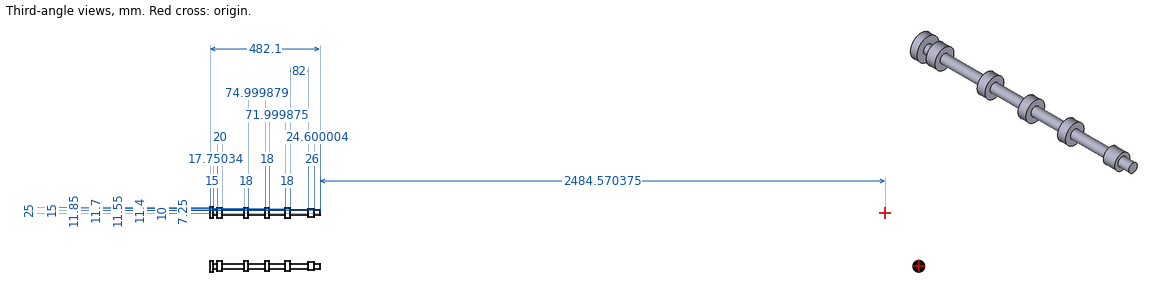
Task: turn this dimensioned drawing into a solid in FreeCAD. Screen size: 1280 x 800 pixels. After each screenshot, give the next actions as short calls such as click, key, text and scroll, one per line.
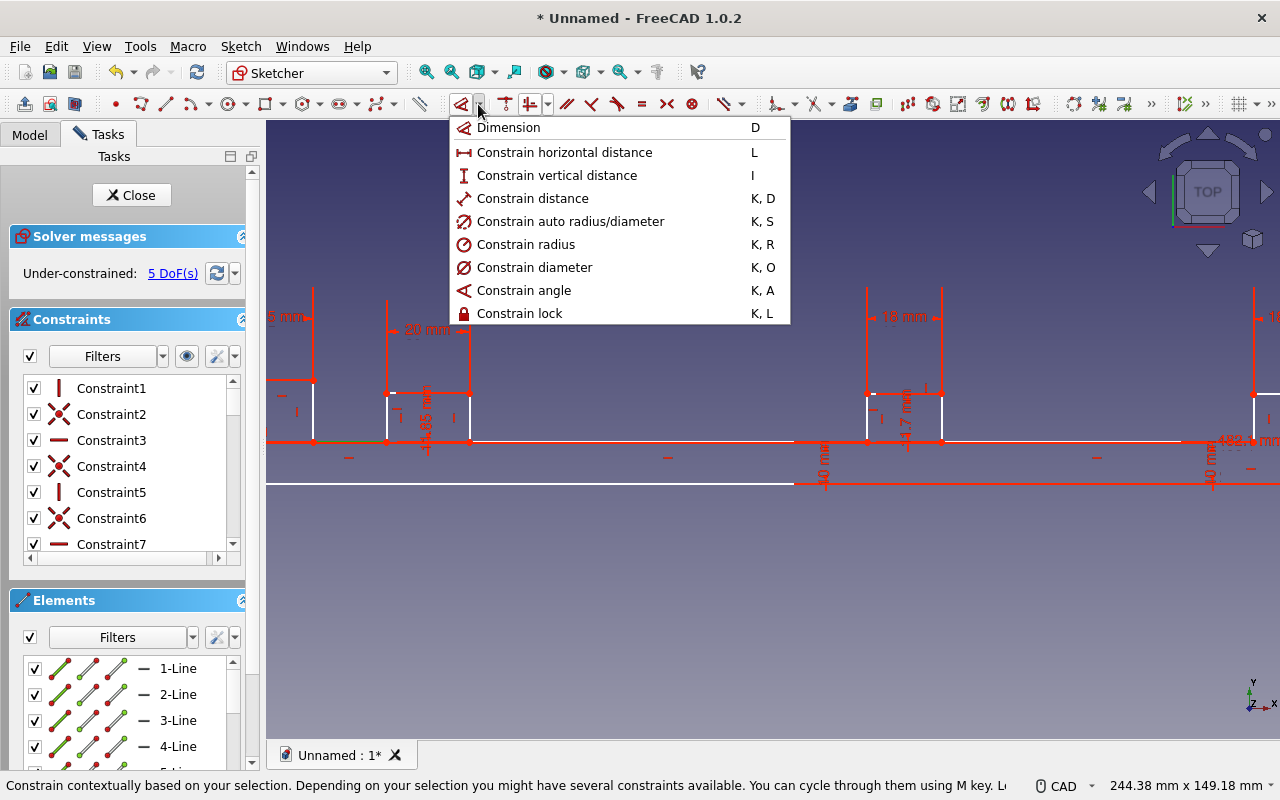
click(620, 152)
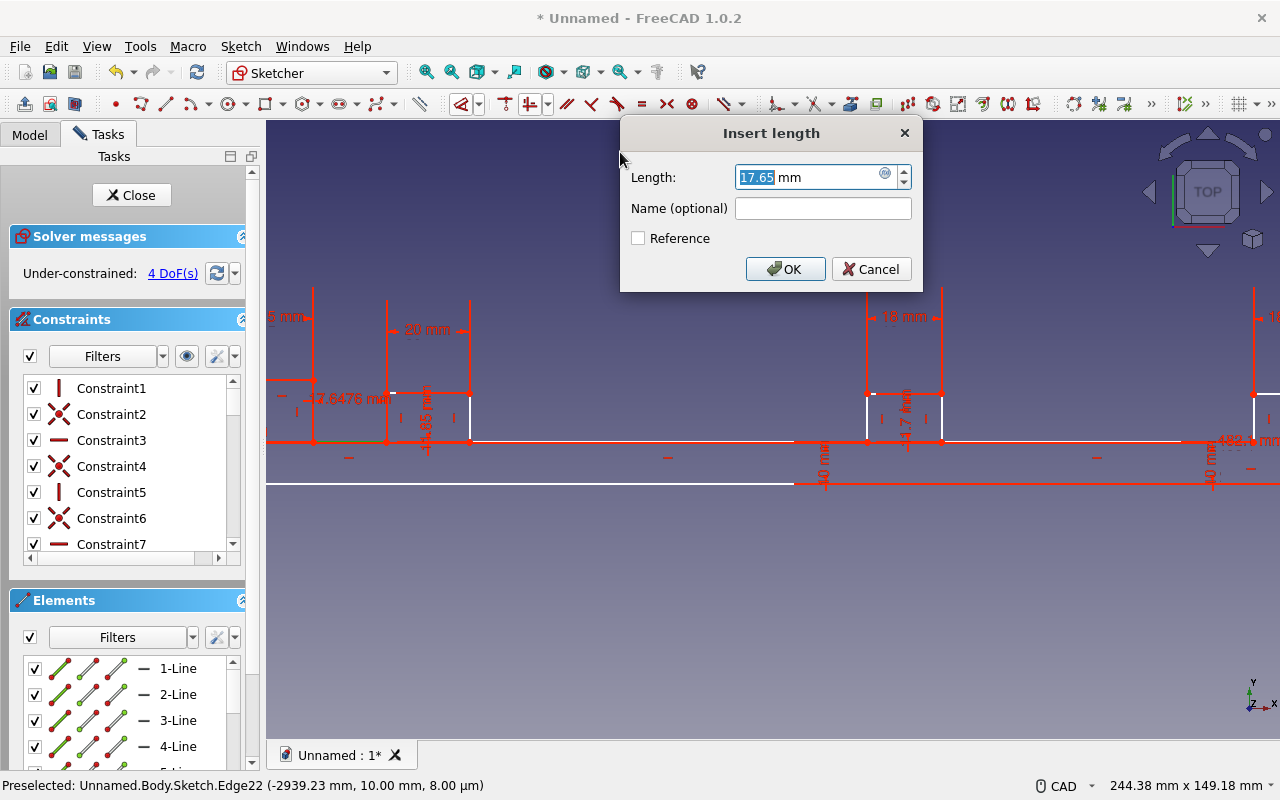
text(17.75034)
key(Return)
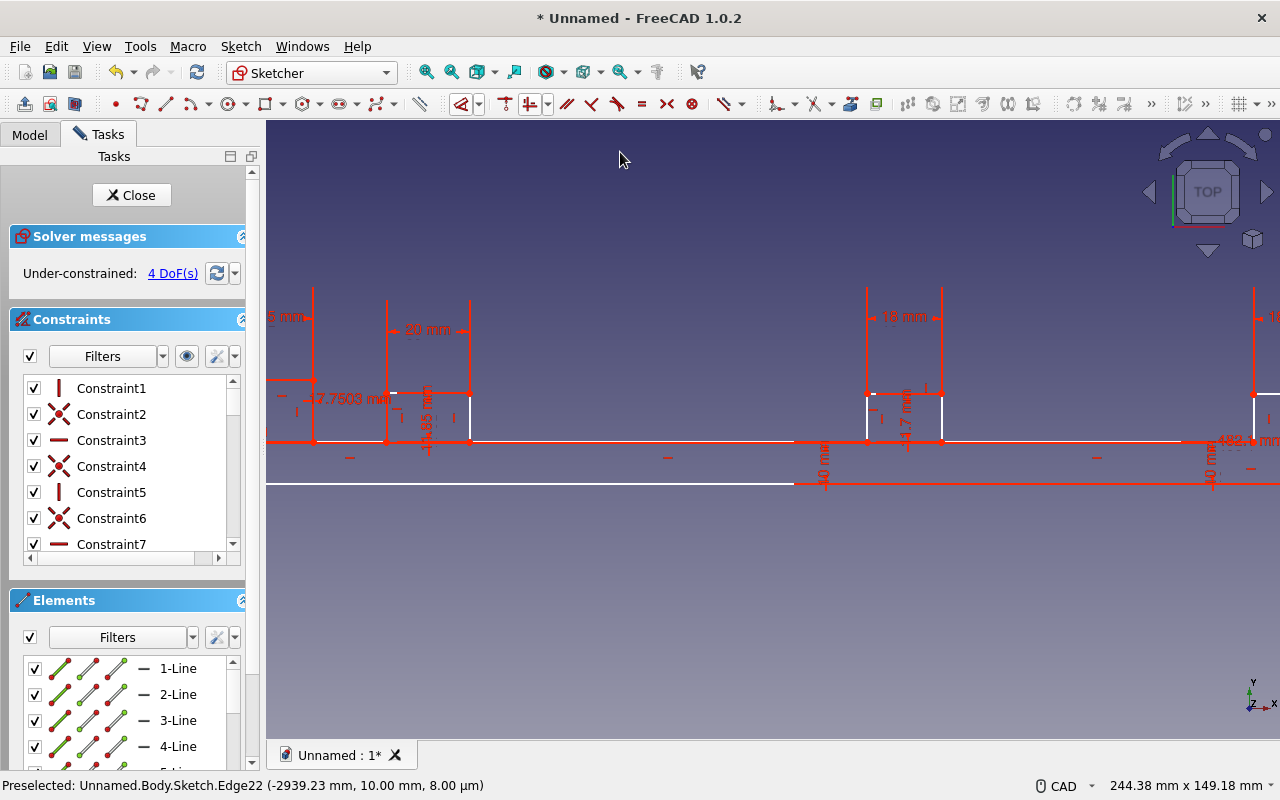
scroll(469, 428, down, 6)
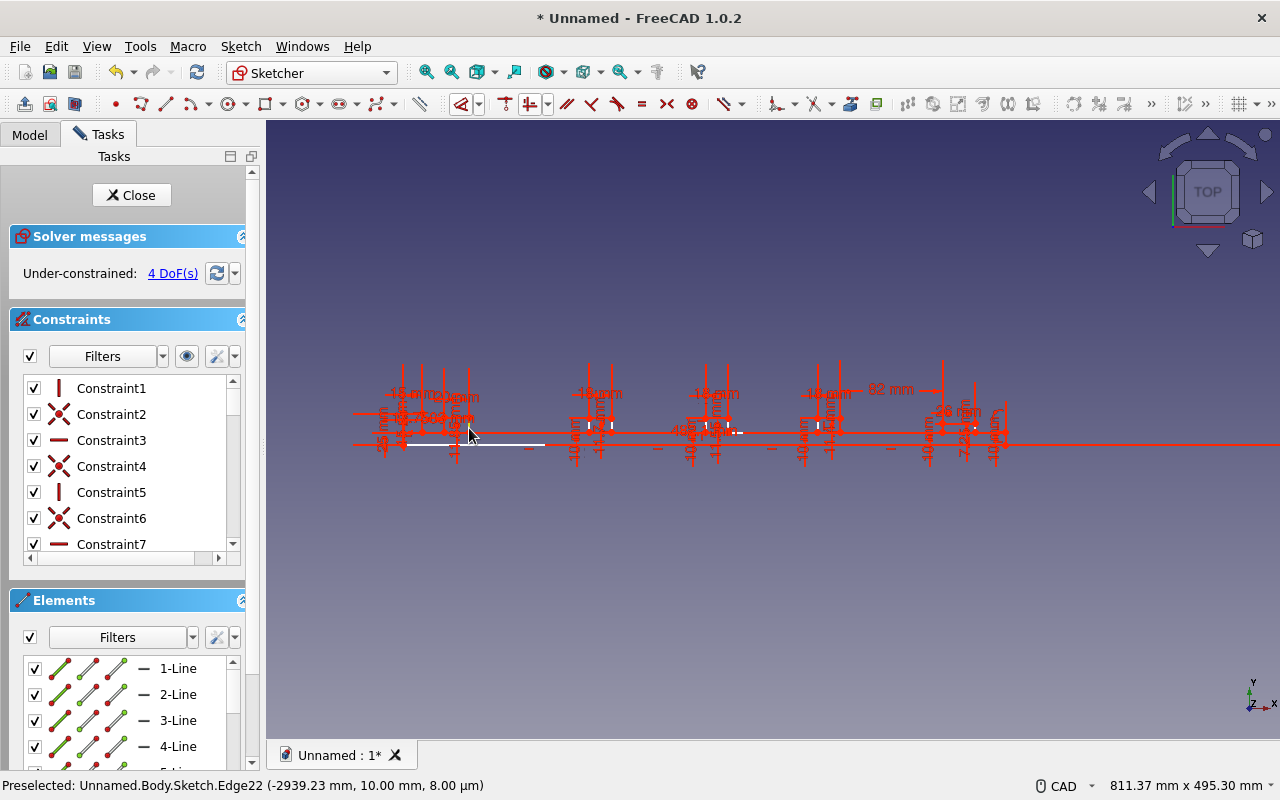
scroll(997, 433, up, 3)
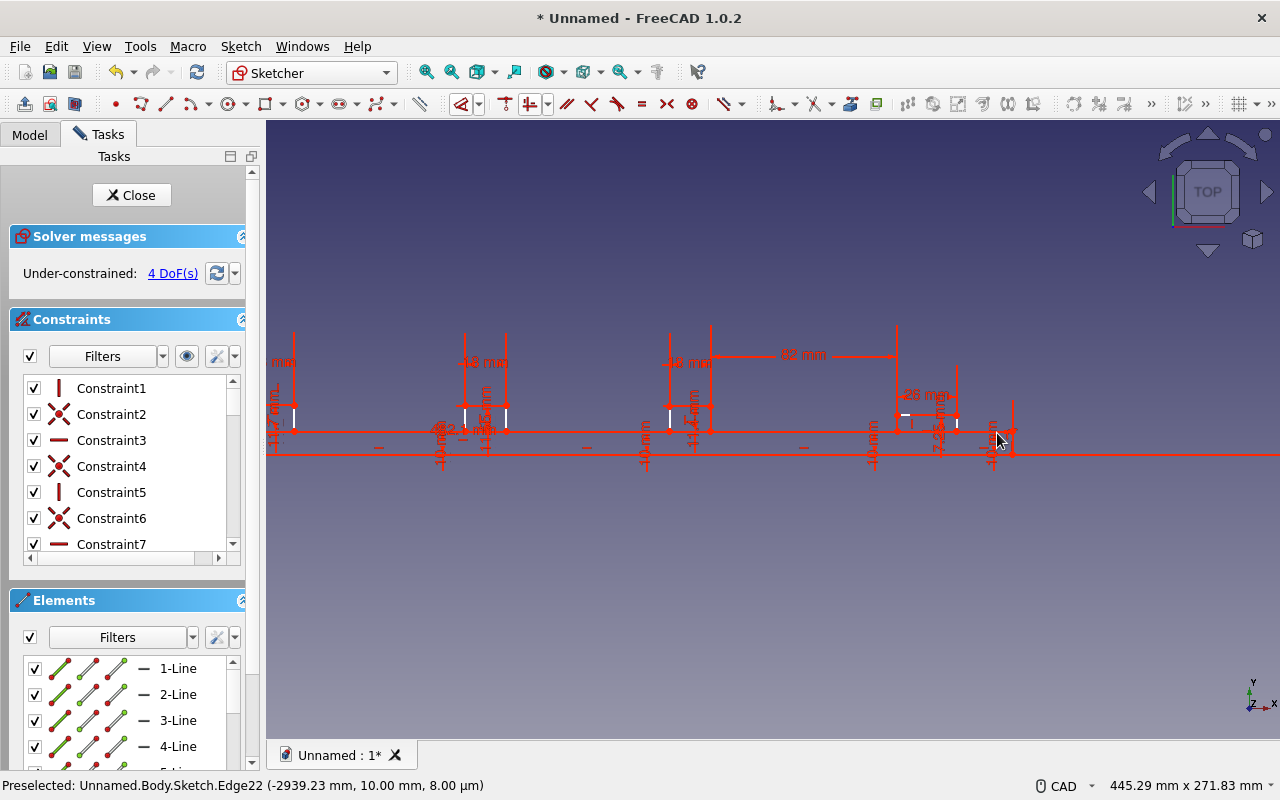
click(973, 432)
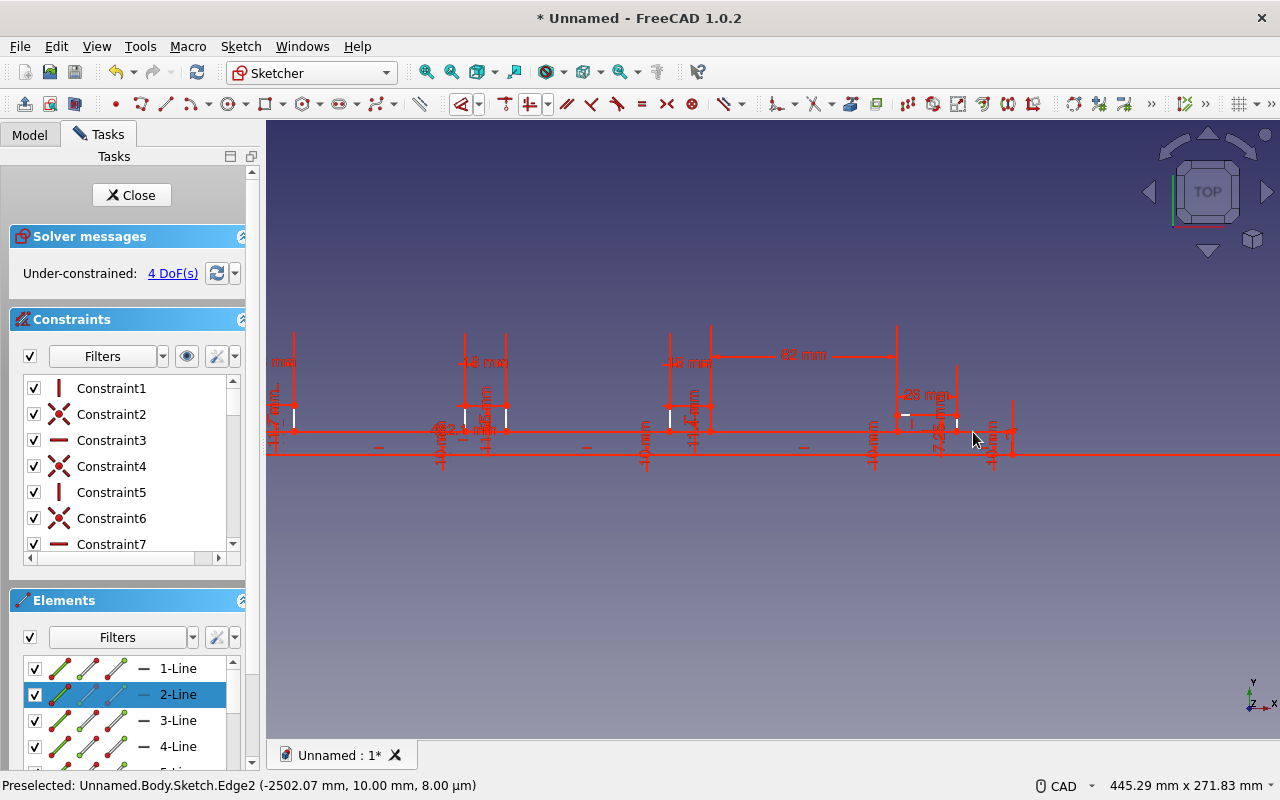
click(478, 104)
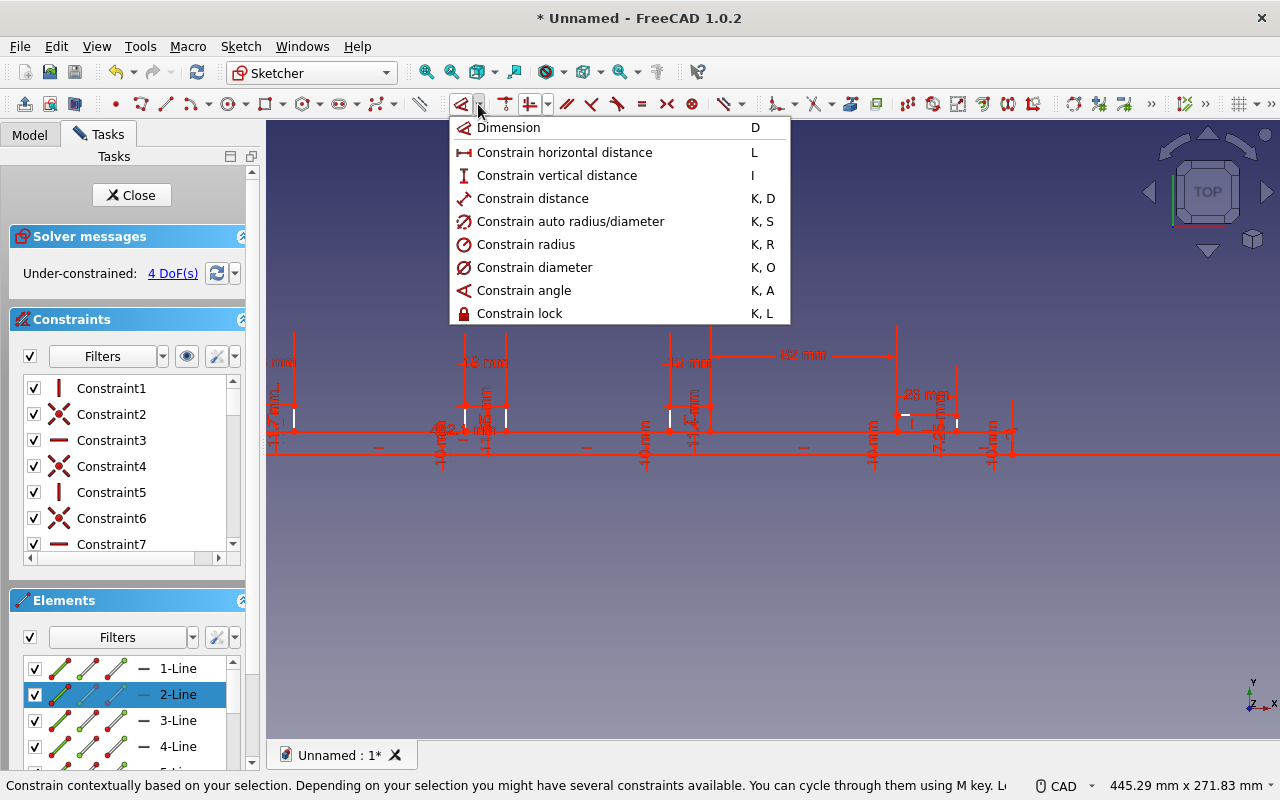
click(620, 152)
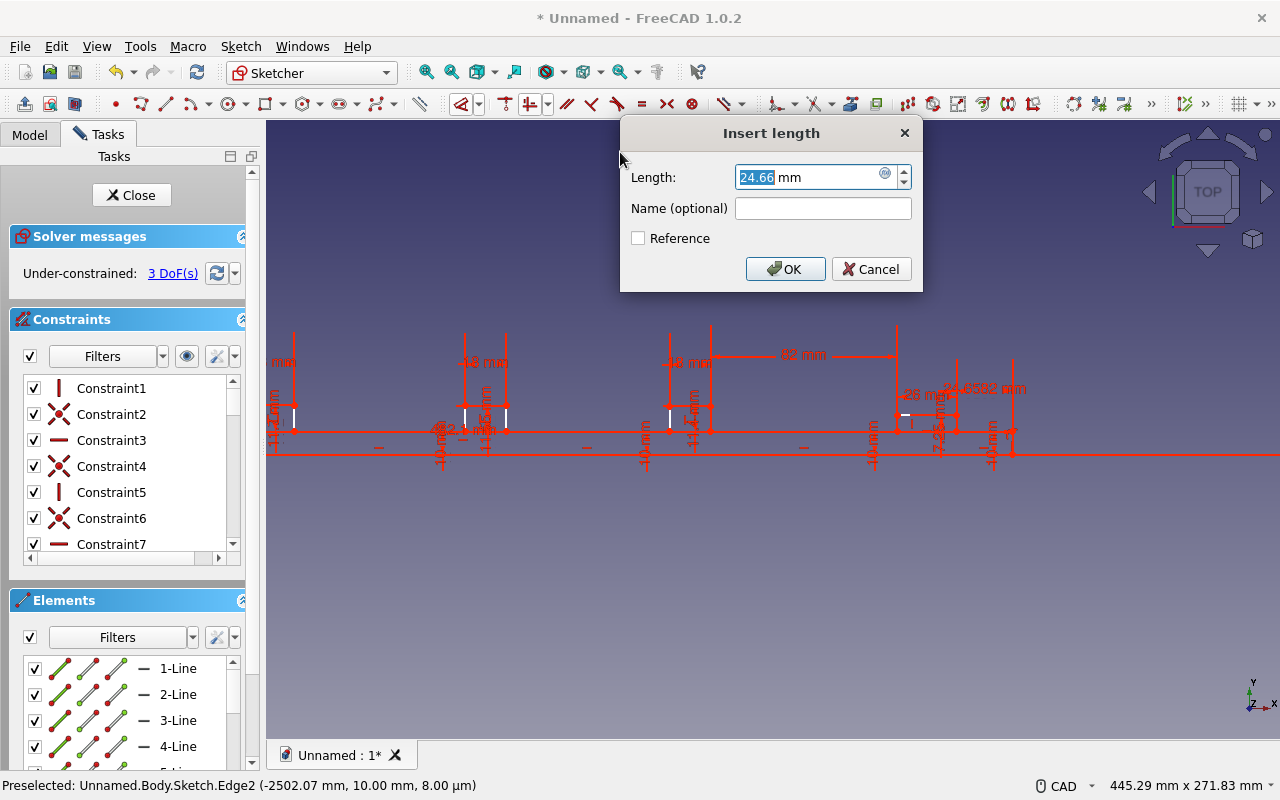
text(24.600004)
key(Return)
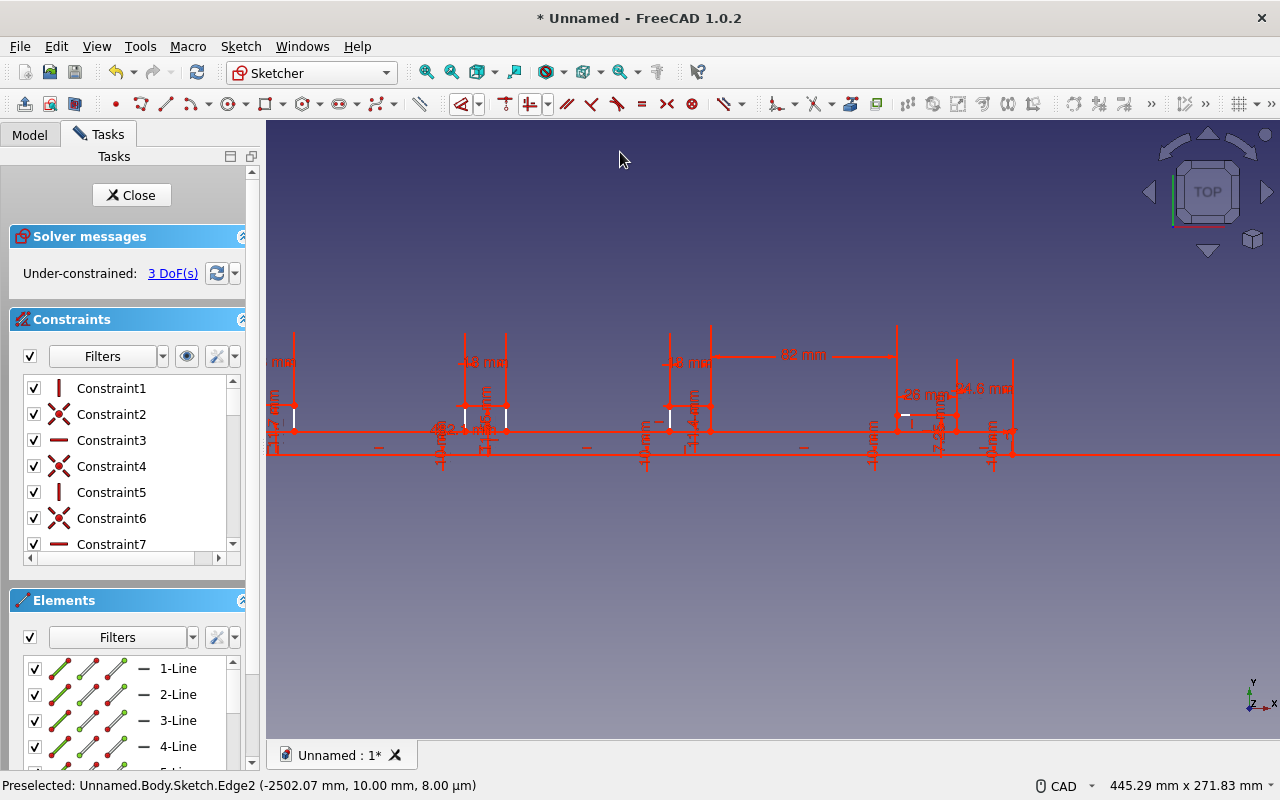
click(621, 432)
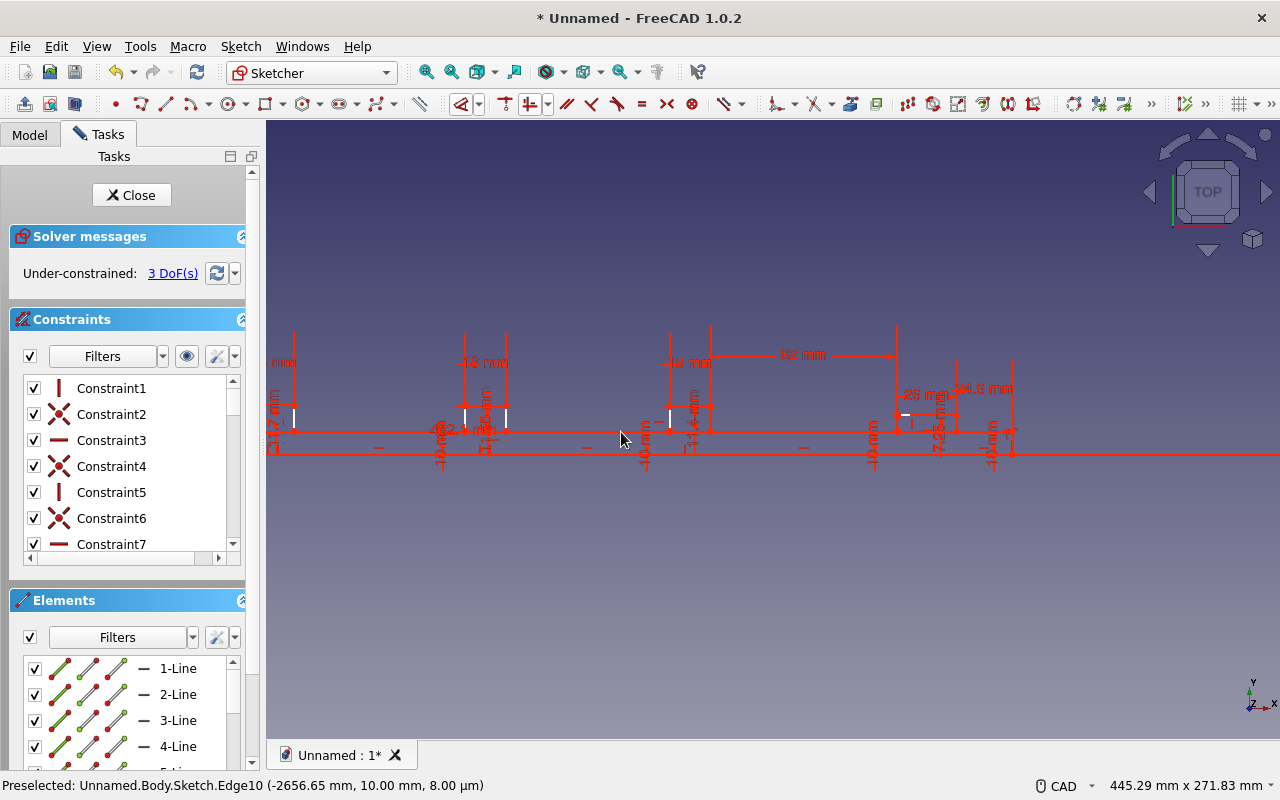
click(478, 104)